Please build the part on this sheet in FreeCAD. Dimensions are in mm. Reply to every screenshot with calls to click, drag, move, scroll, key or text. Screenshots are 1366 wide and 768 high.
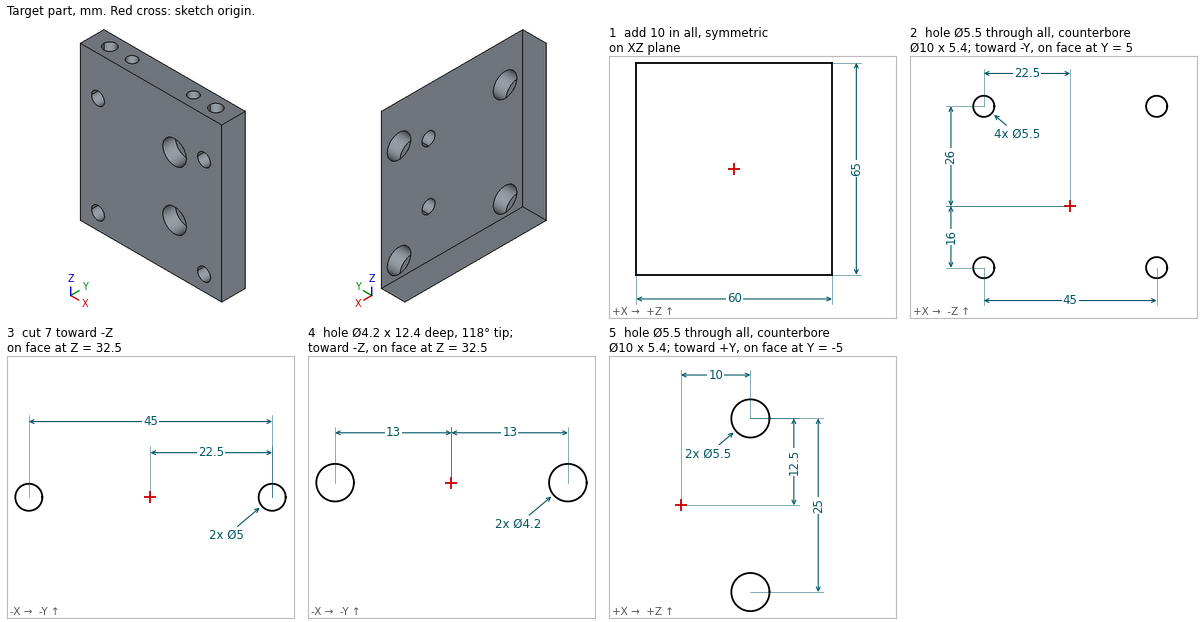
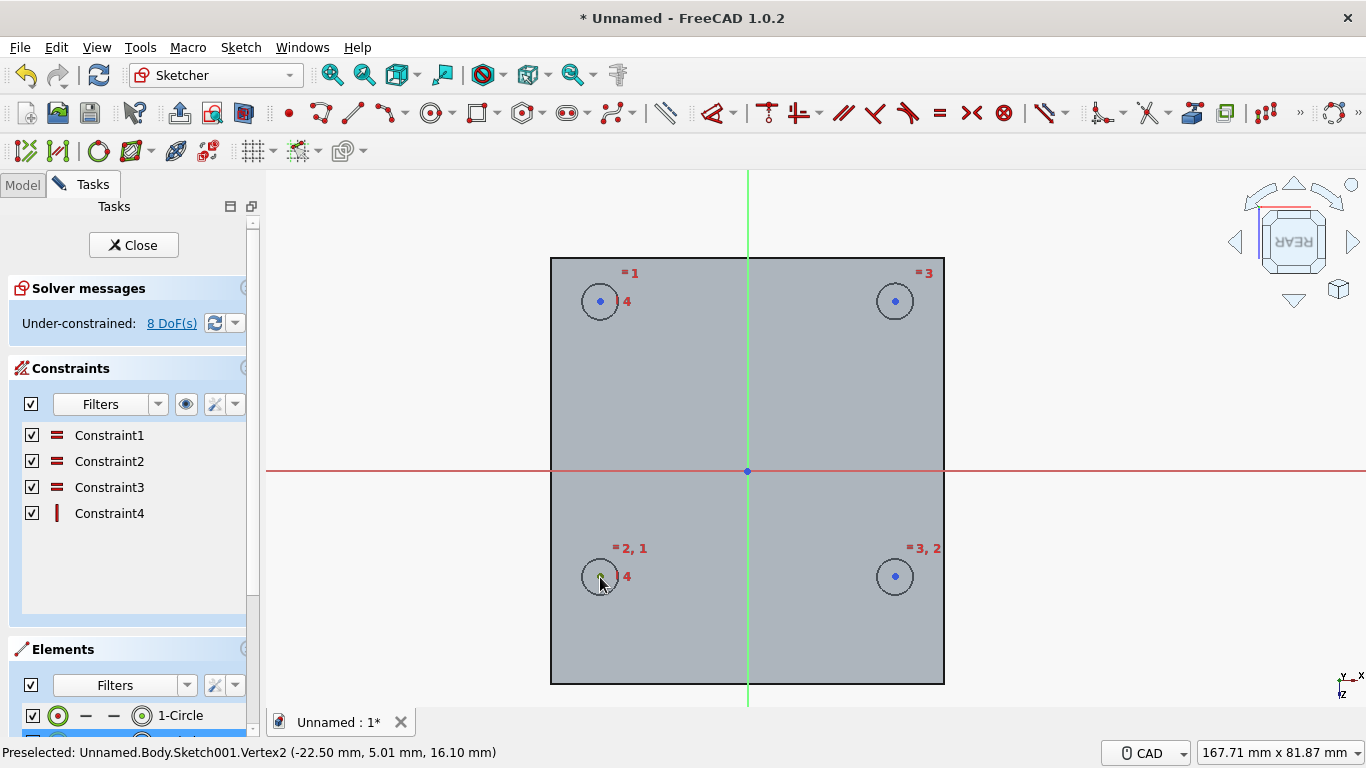
click(895, 577)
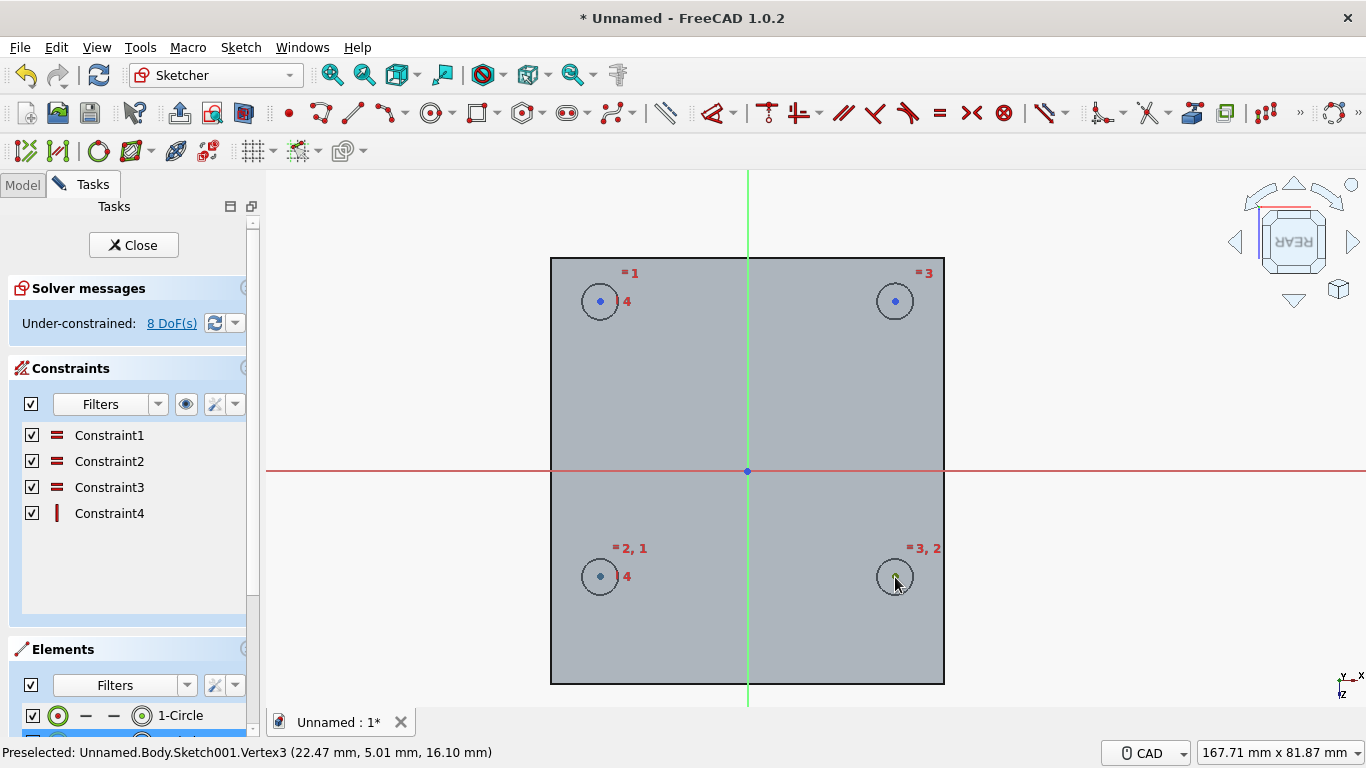
click(822, 114)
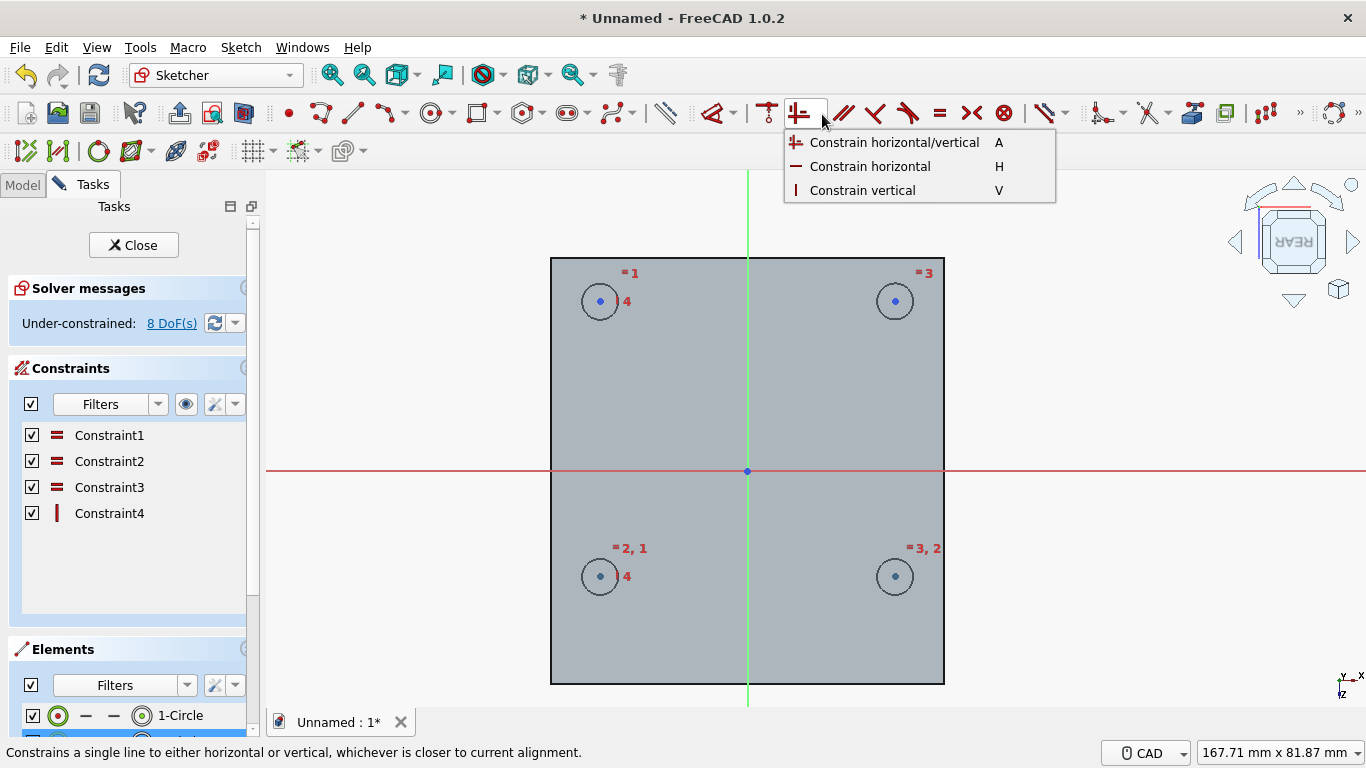
click(920, 166)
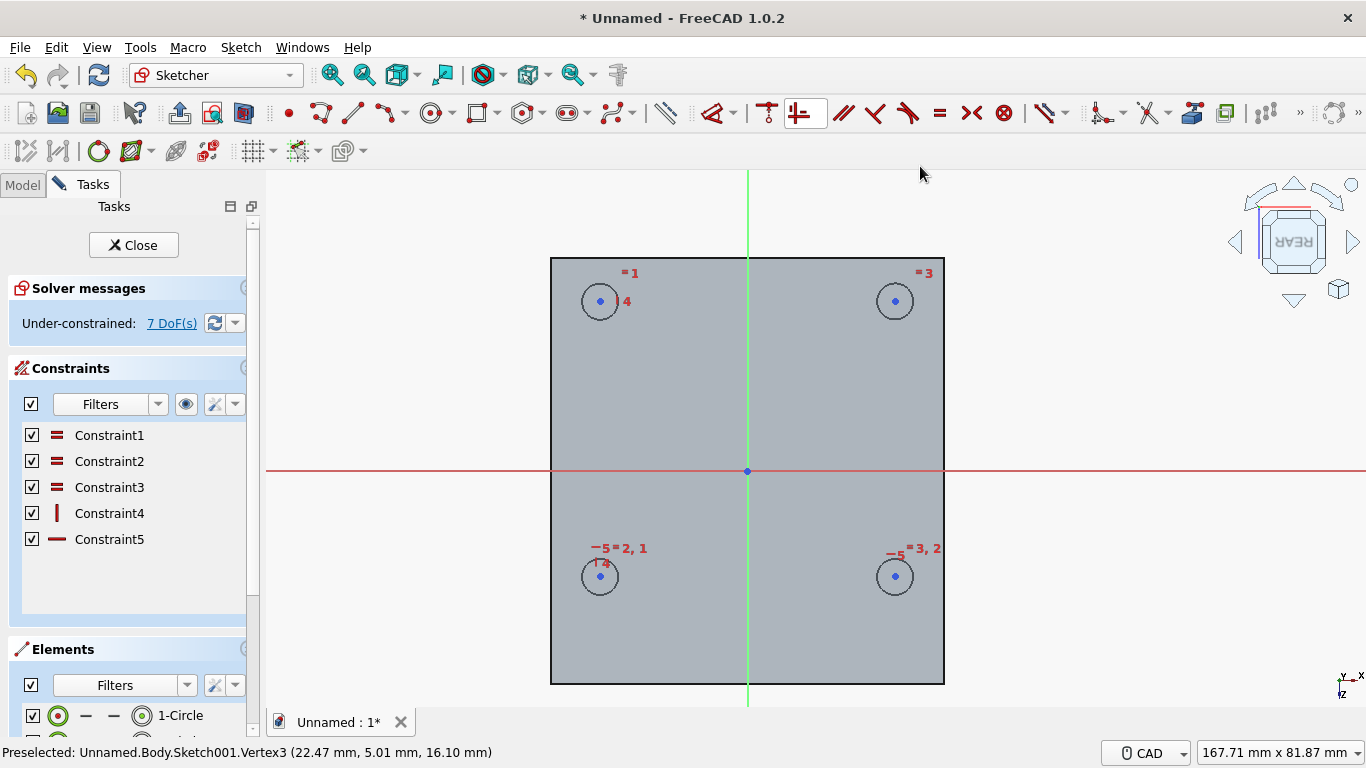
click(895, 577)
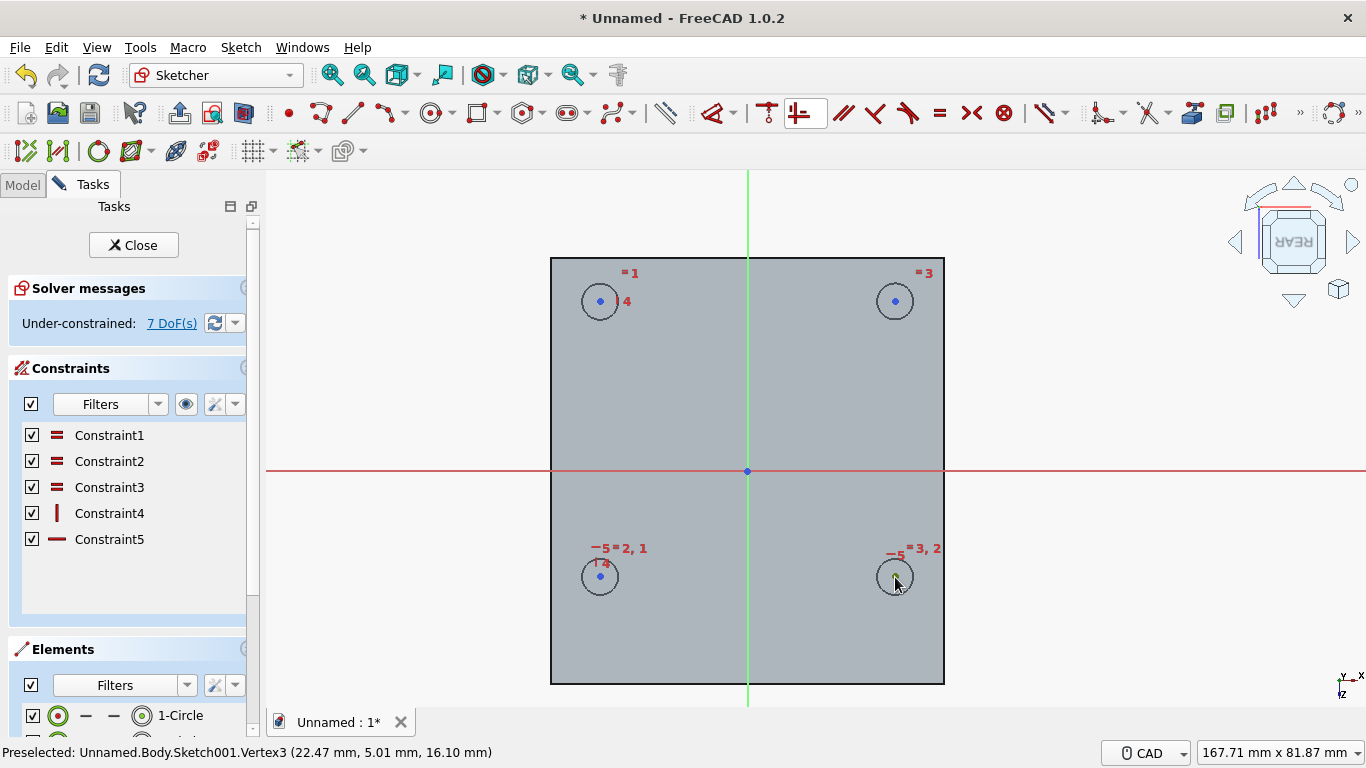
click(895, 301)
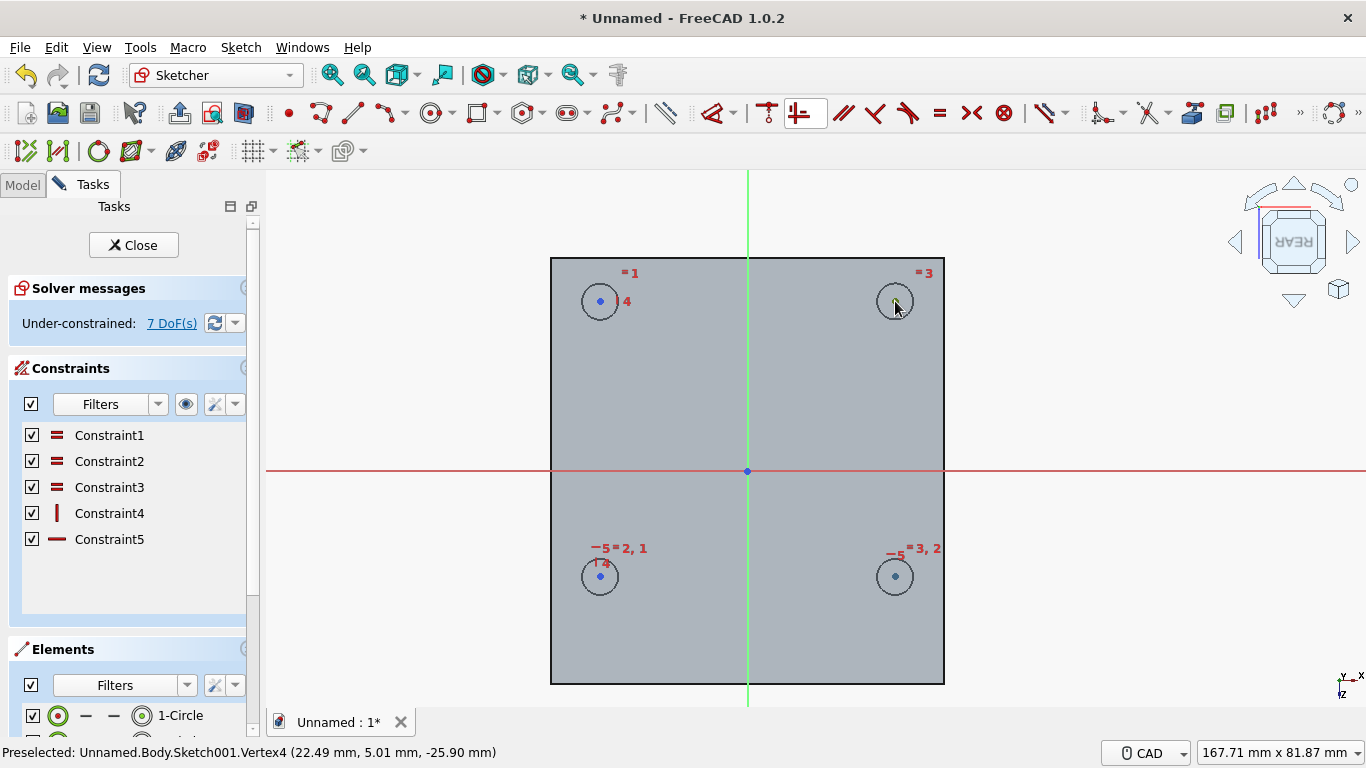
key(v)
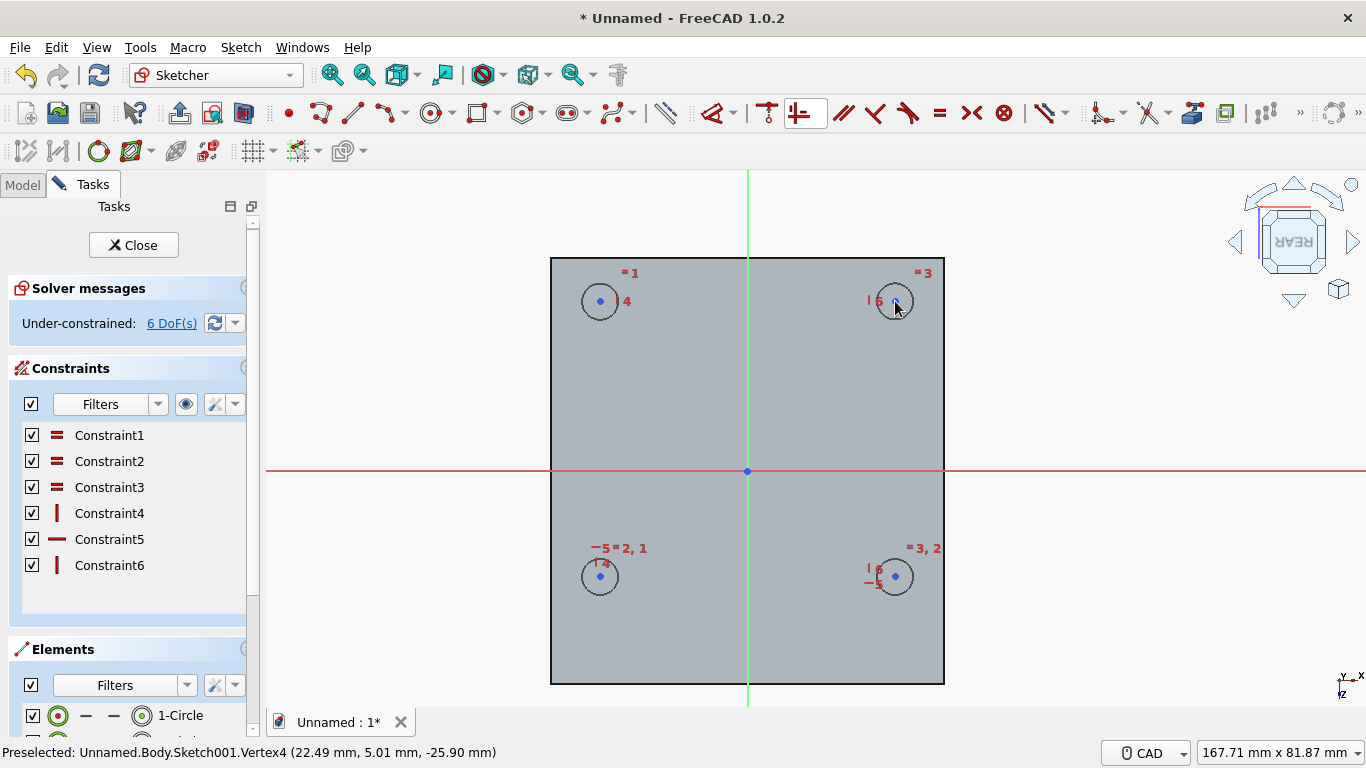
click(600, 302)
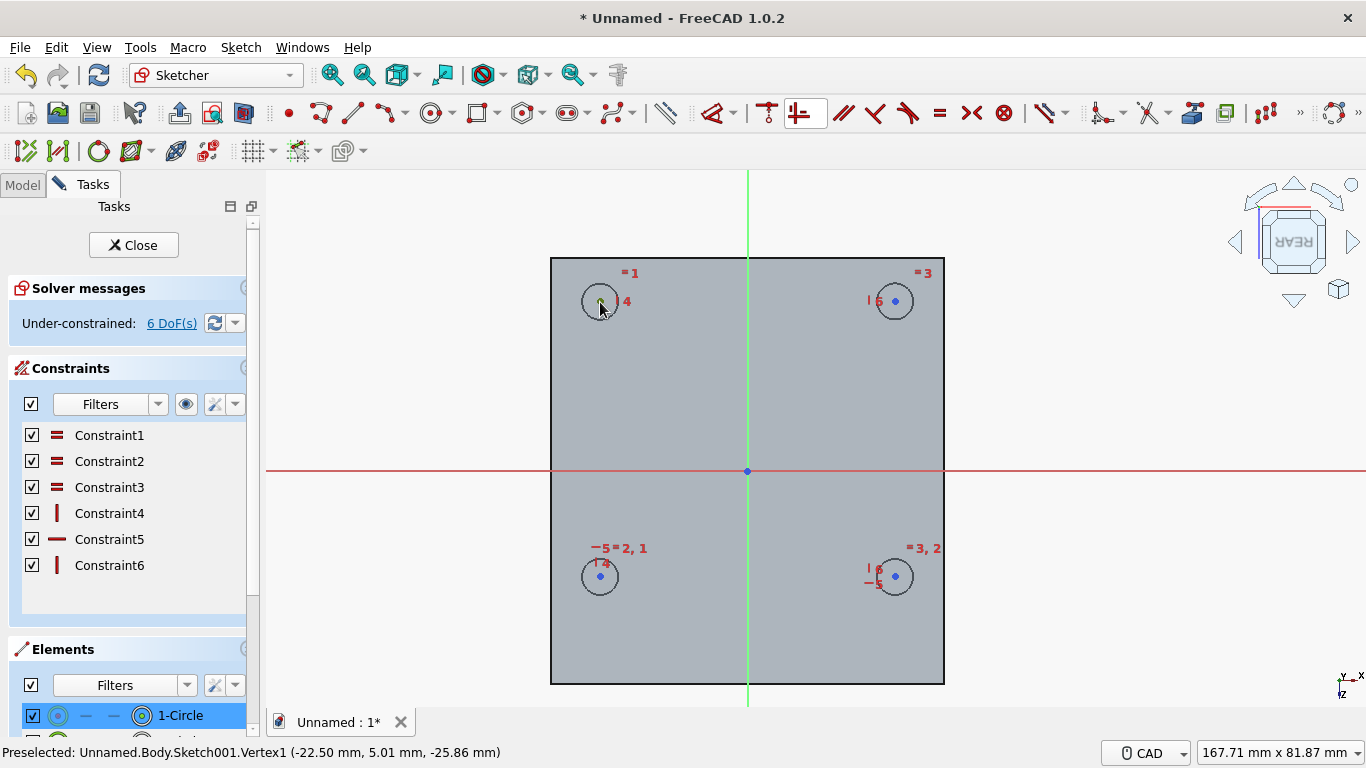
click(895, 301)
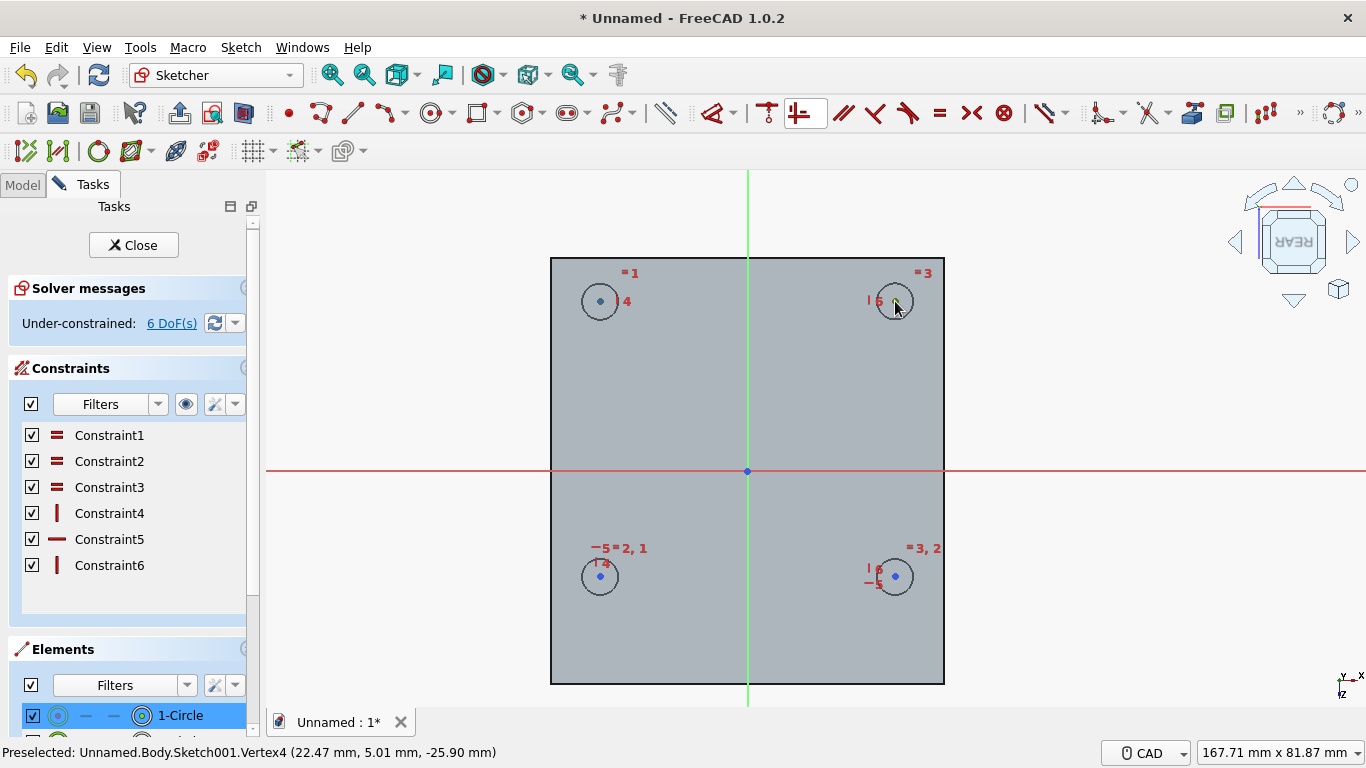
key(h)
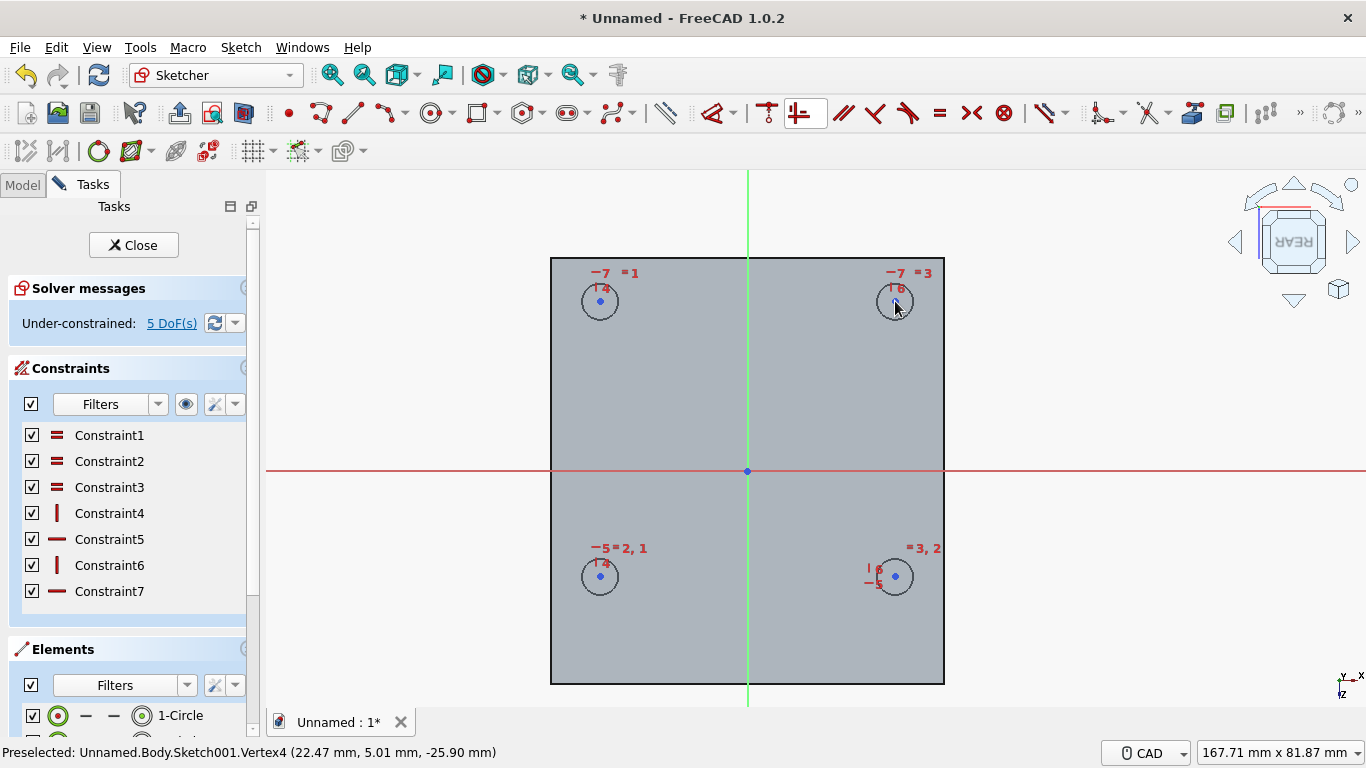
click(613, 289)